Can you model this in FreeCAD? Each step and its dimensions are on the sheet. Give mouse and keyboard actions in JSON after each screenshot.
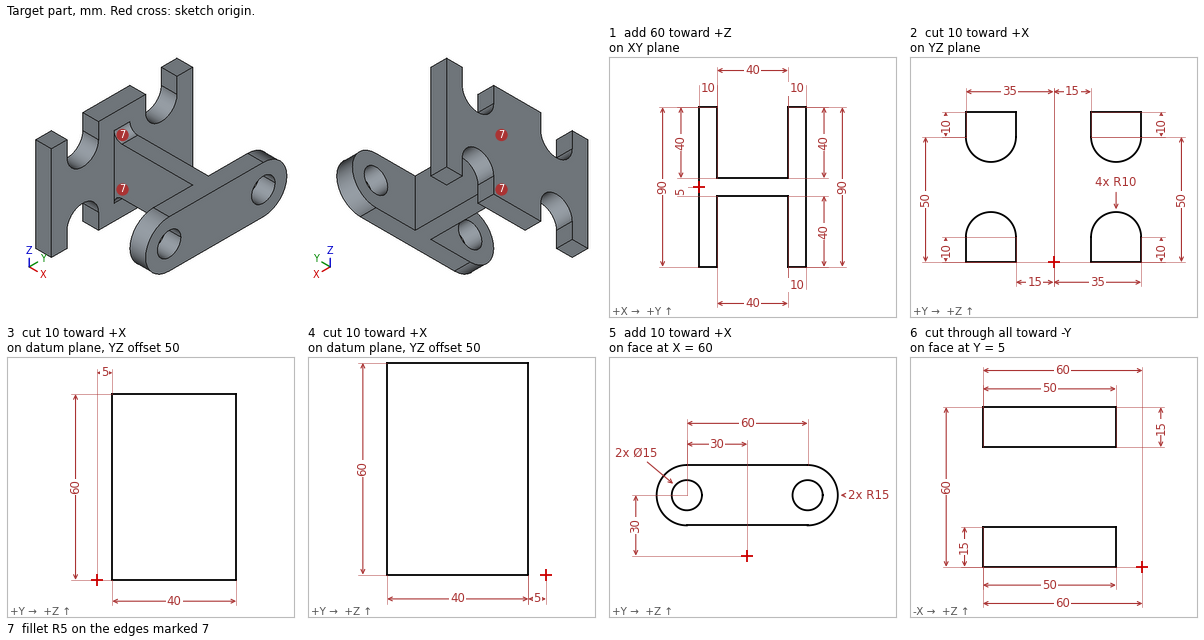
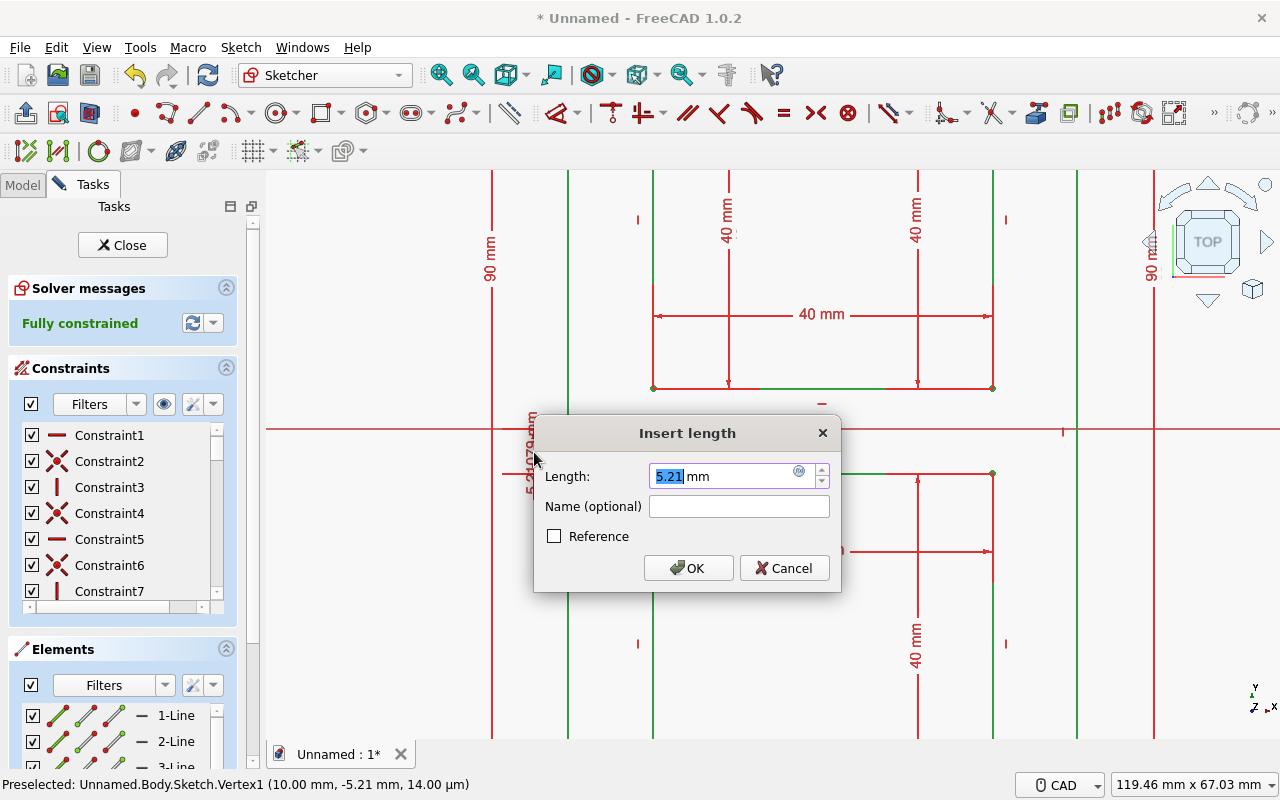
{"action": "type", "text": "5"}
{"action": "key", "text": "Return"}
{"action": "key", "text": "Escape"}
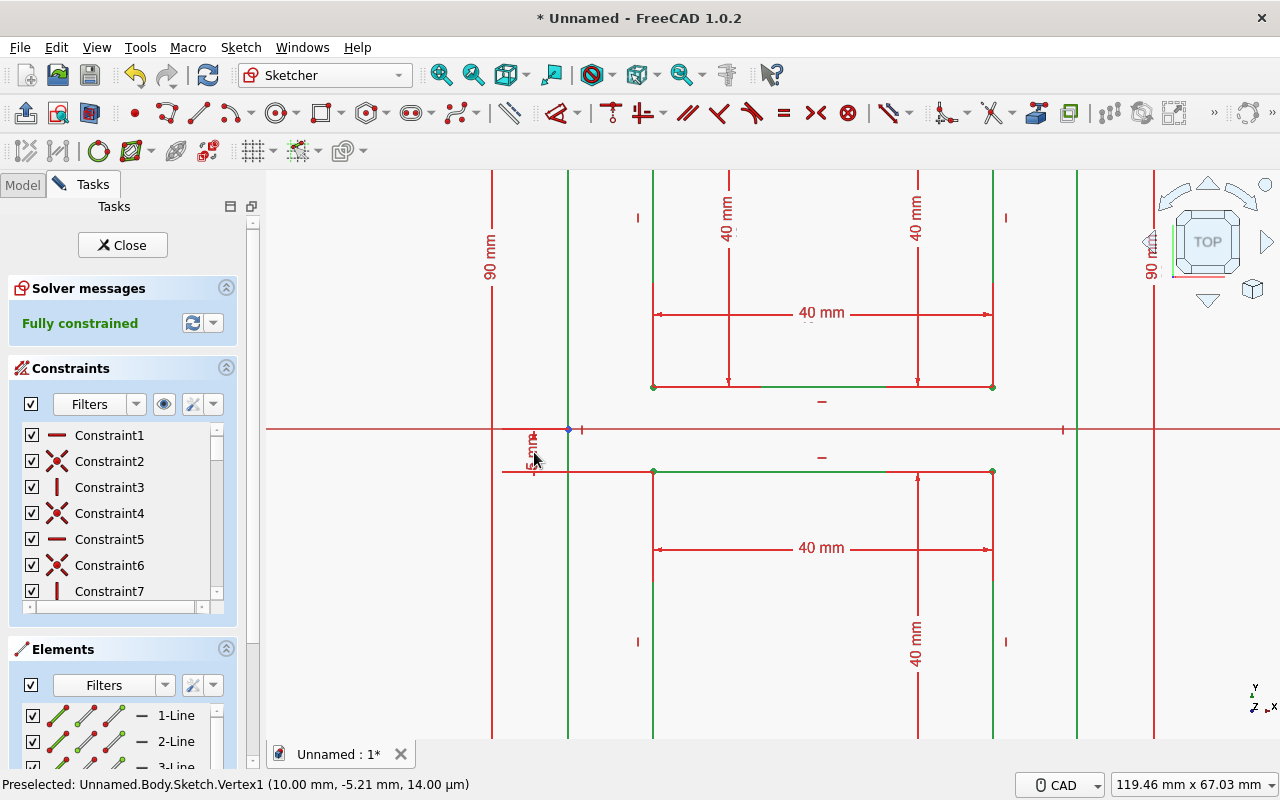
{"action": "left_click", "coordinate": [123, 245]}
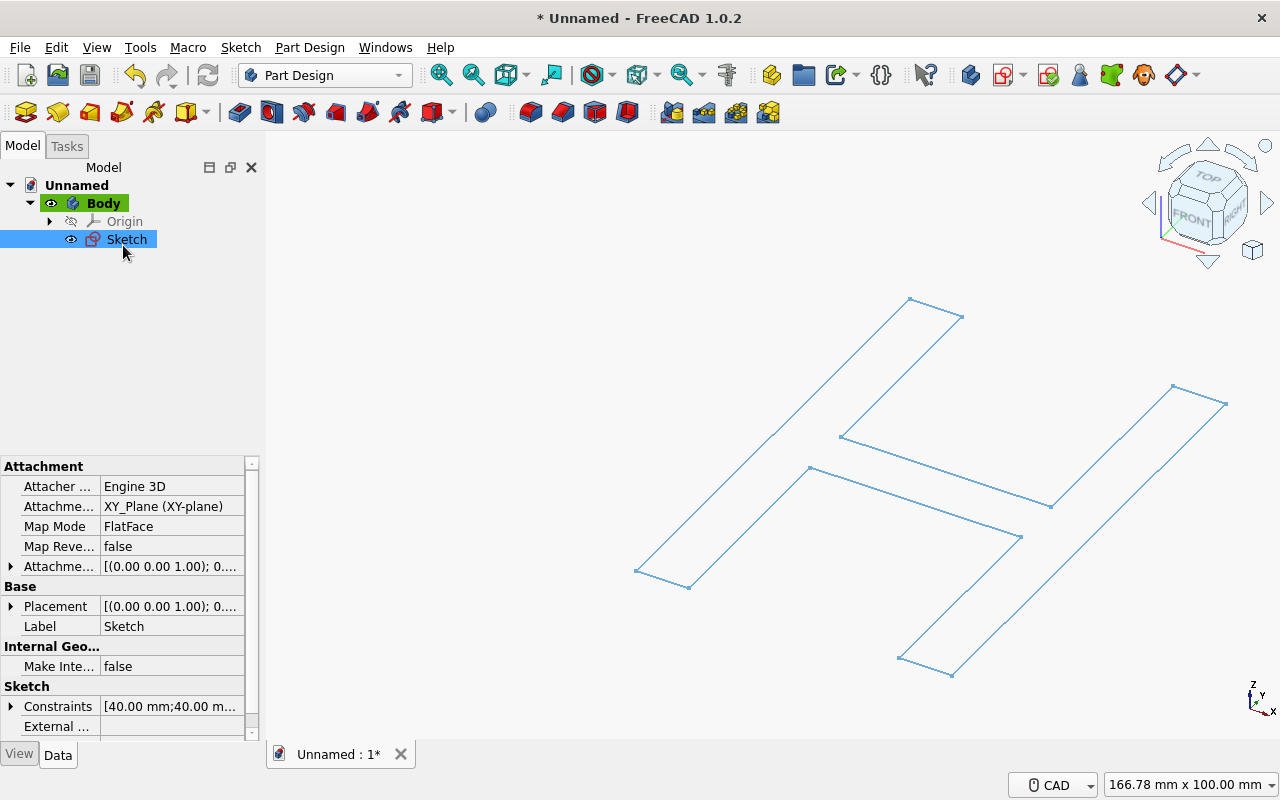
{"action": "left_click", "coordinate": [26, 112]}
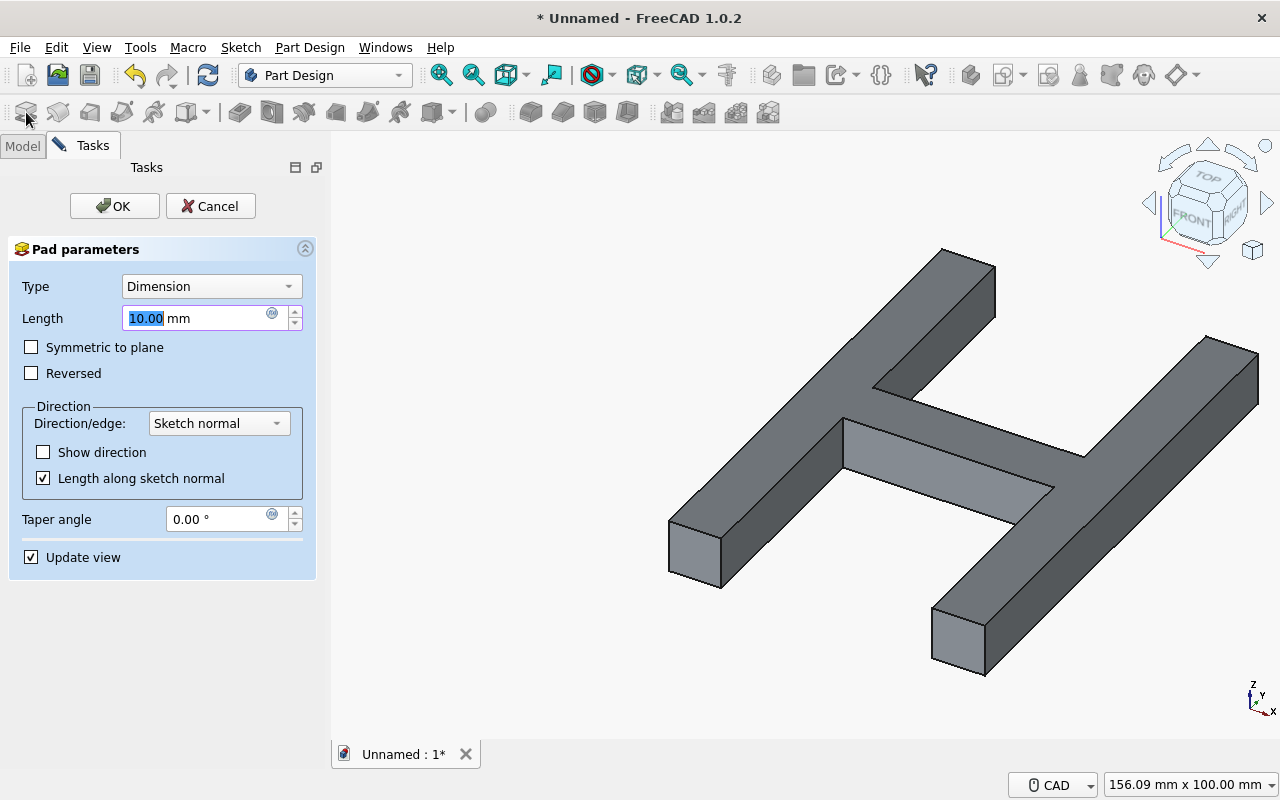
{"action": "type", "text": "60"}
{"action": "key", "text": "Tab"}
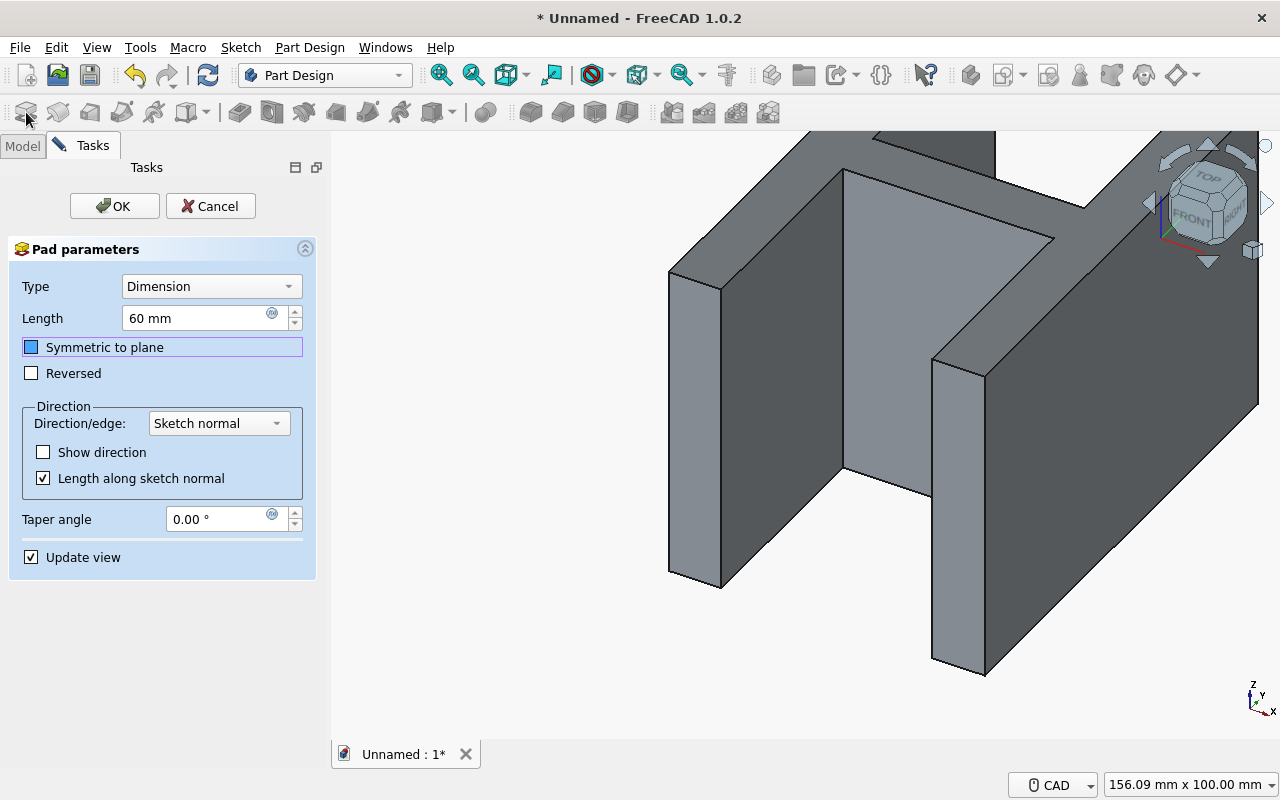
{"action": "left_click", "coordinate": [115, 206]}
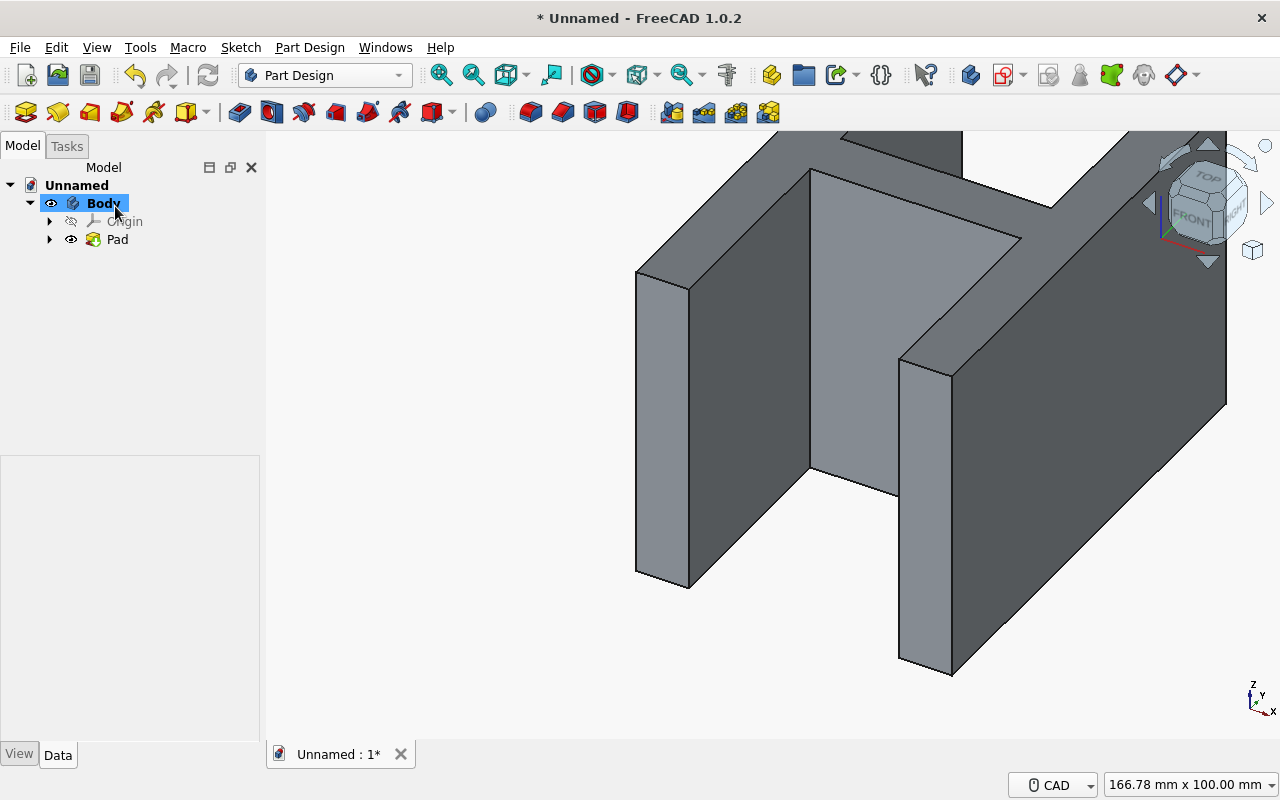
{"action": "left_click", "coordinate": [442, 76]}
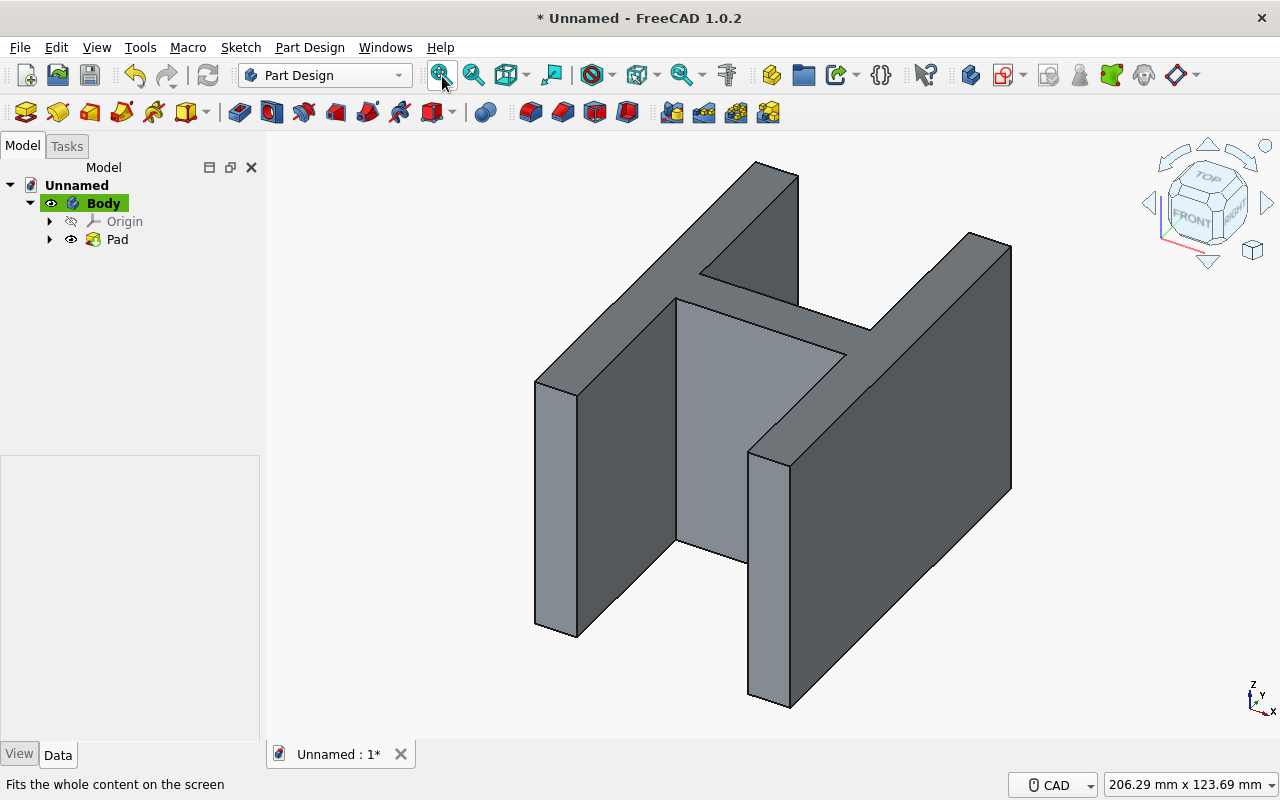
{"action": "left_click", "coordinate": [1004, 76]}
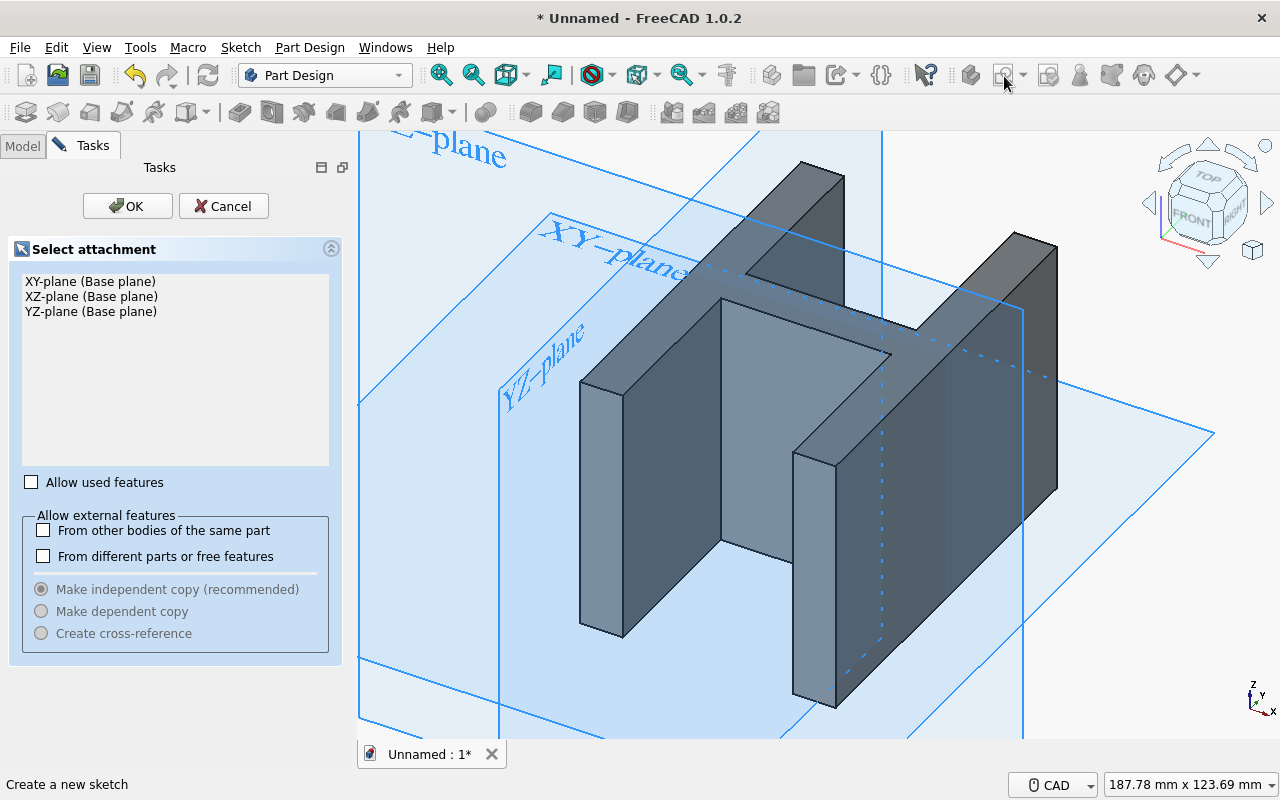
{"action": "left_click", "coordinate": [82, 312]}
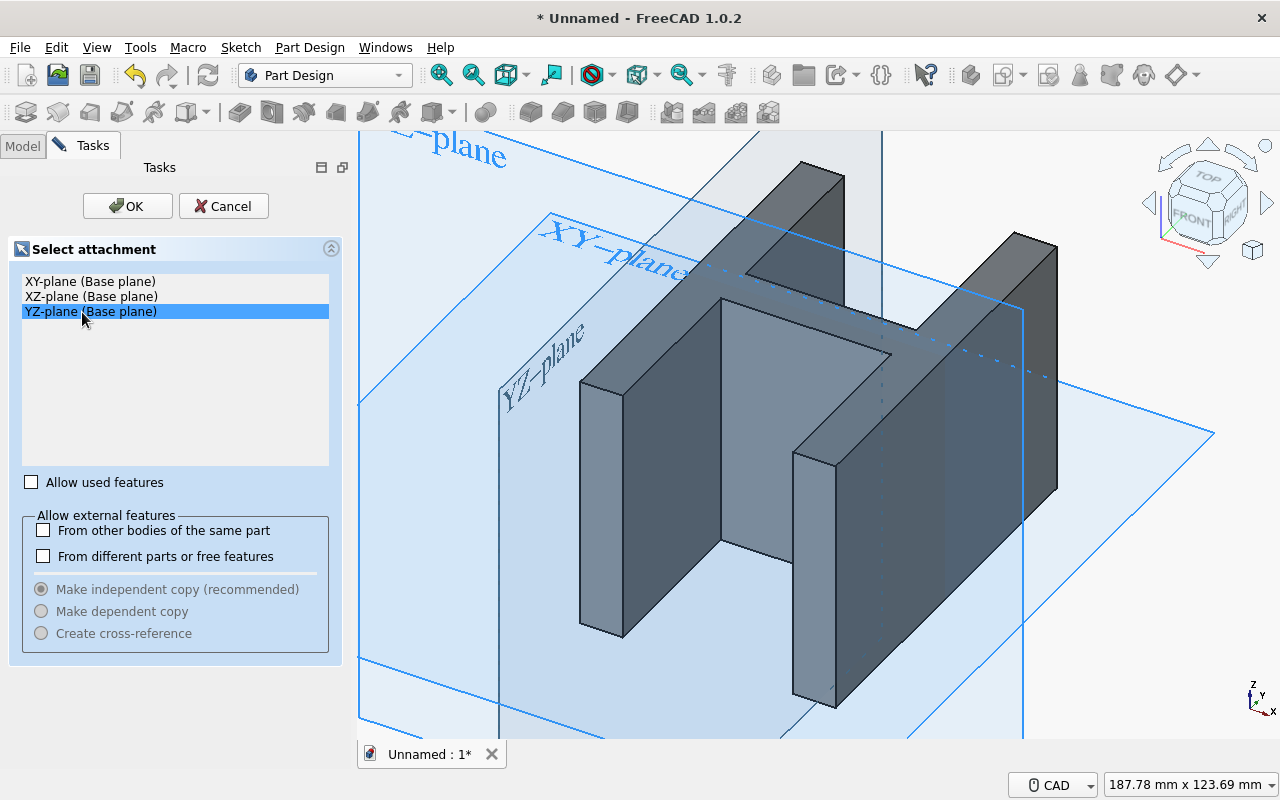
{"action": "left_click", "coordinate": [128, 206]}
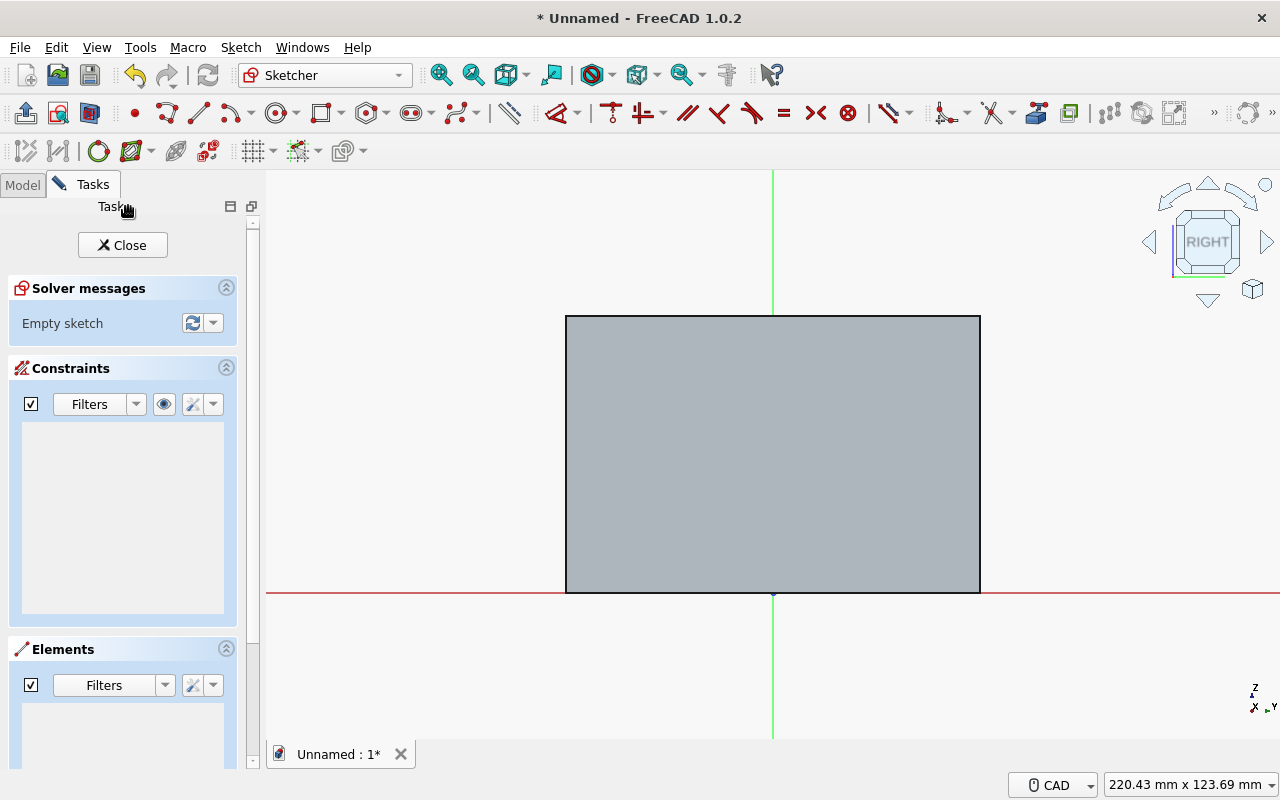
{"action": "left_click", "coordinate": [90, 114]}